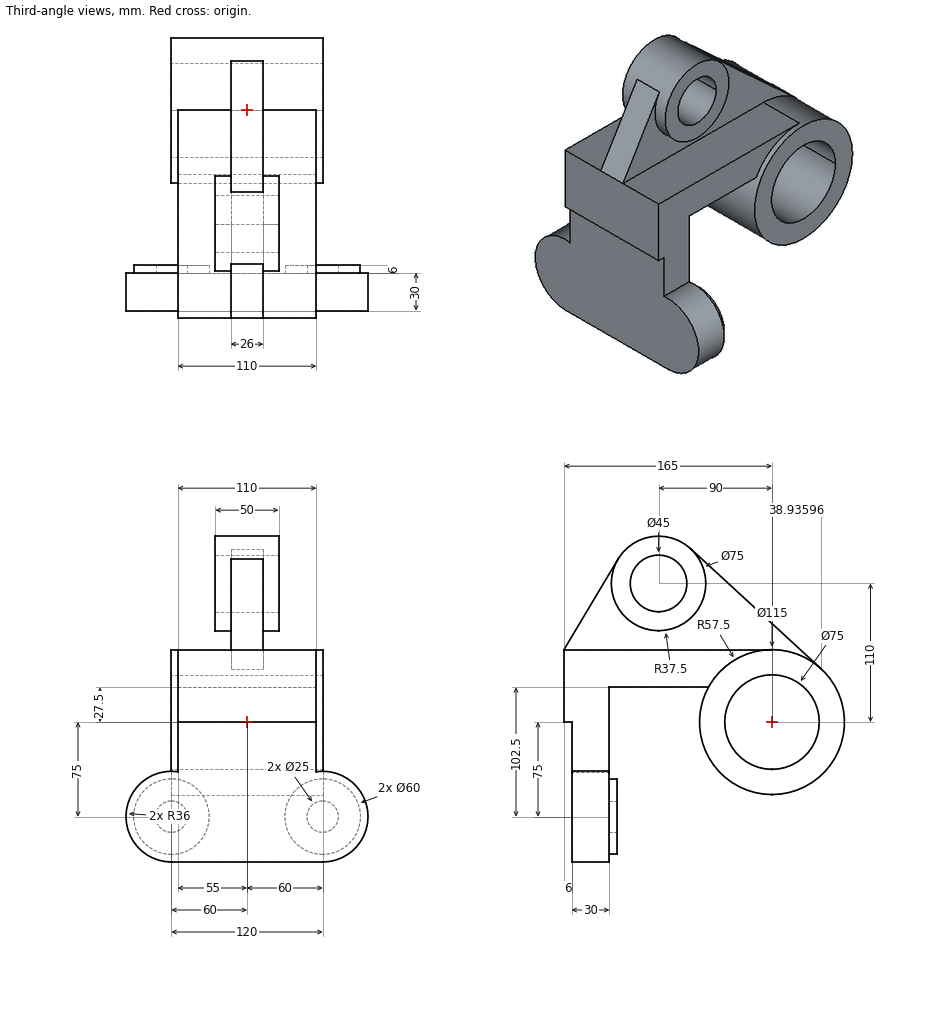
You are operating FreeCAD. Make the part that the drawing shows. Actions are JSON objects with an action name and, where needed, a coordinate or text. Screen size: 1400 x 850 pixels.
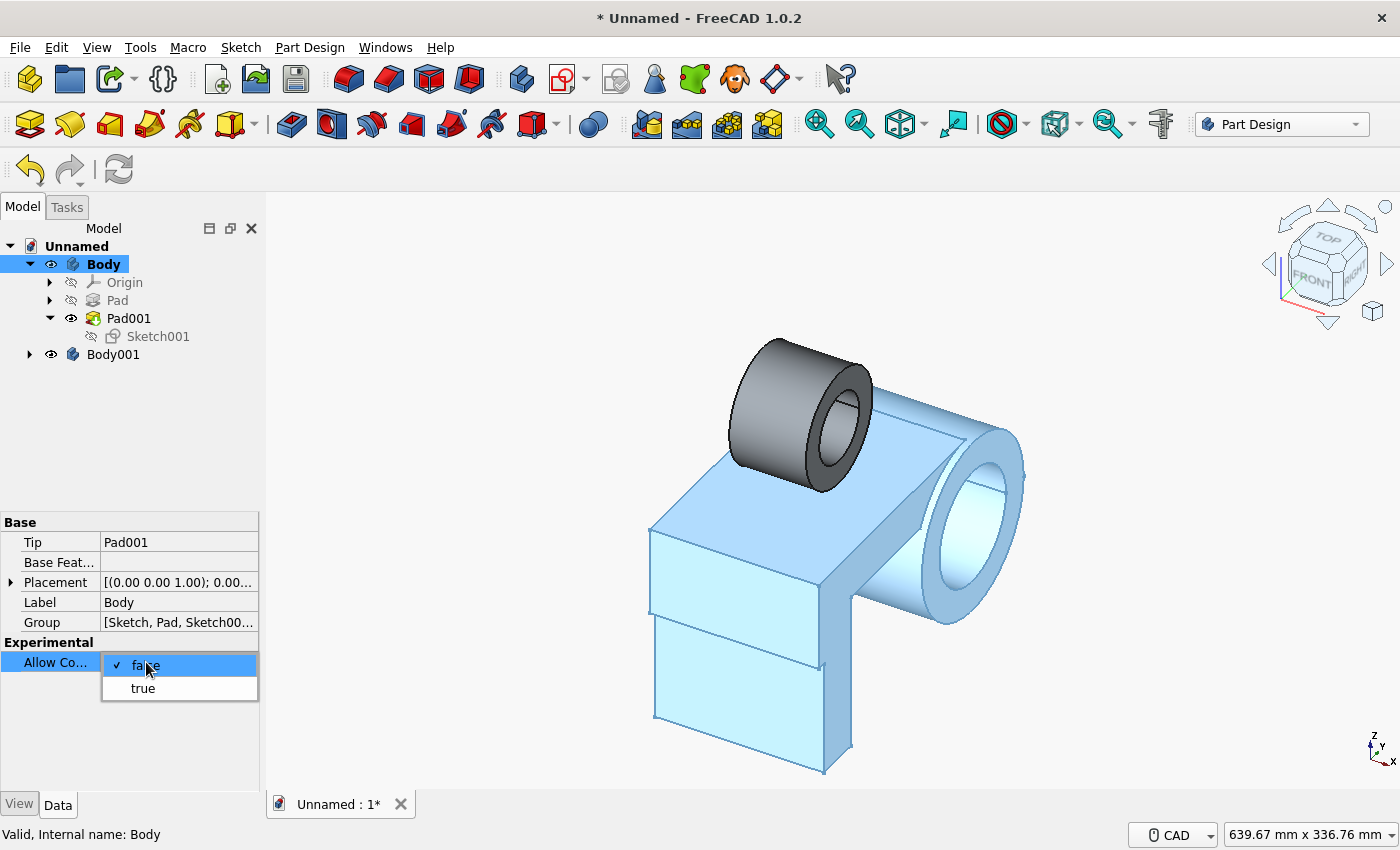
{"action": "left_click", "coordinate": [179, 688]}
{"action": "key", "text": "Return"}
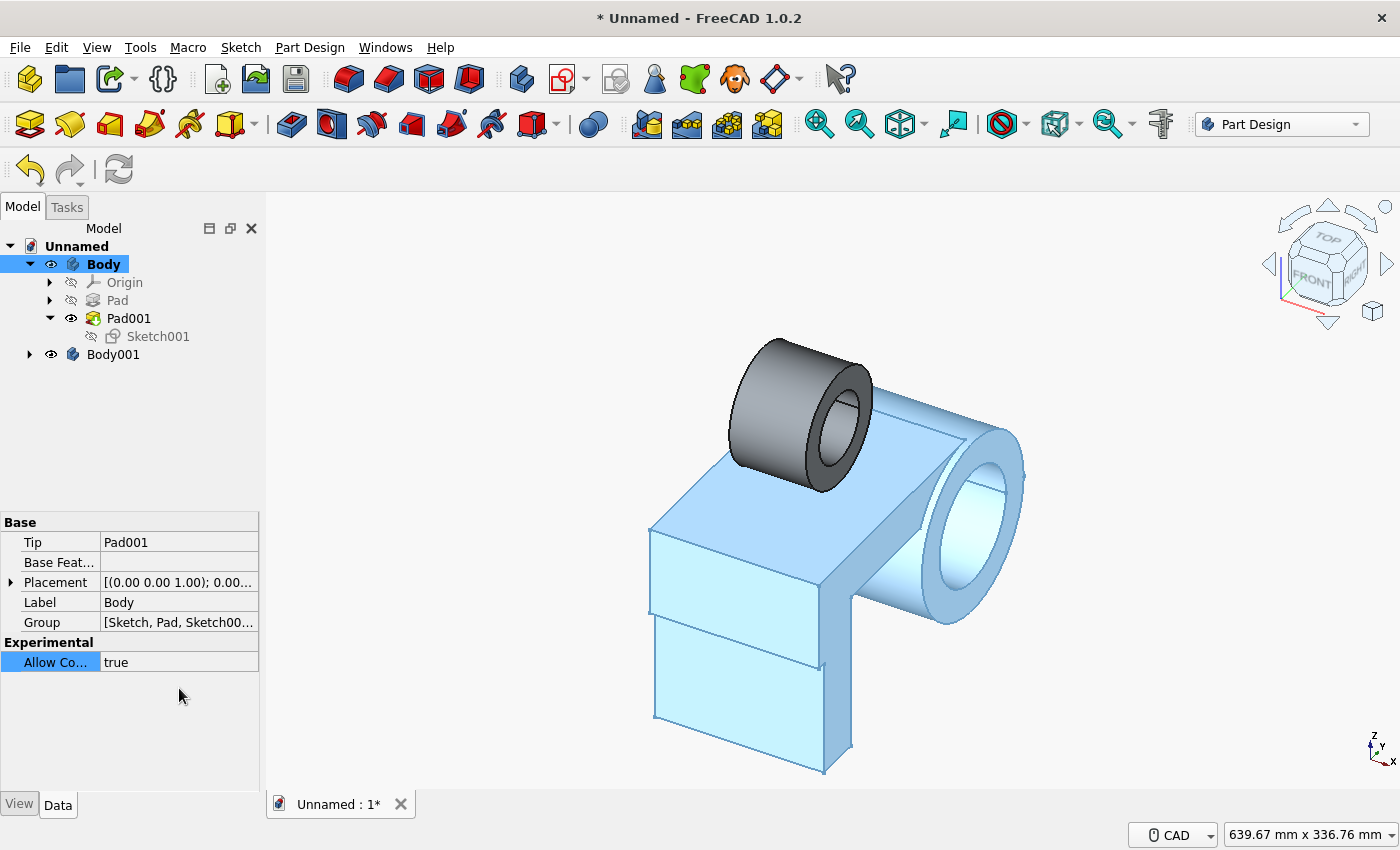
{"action": "left_click", "coordinate": [96, 354]}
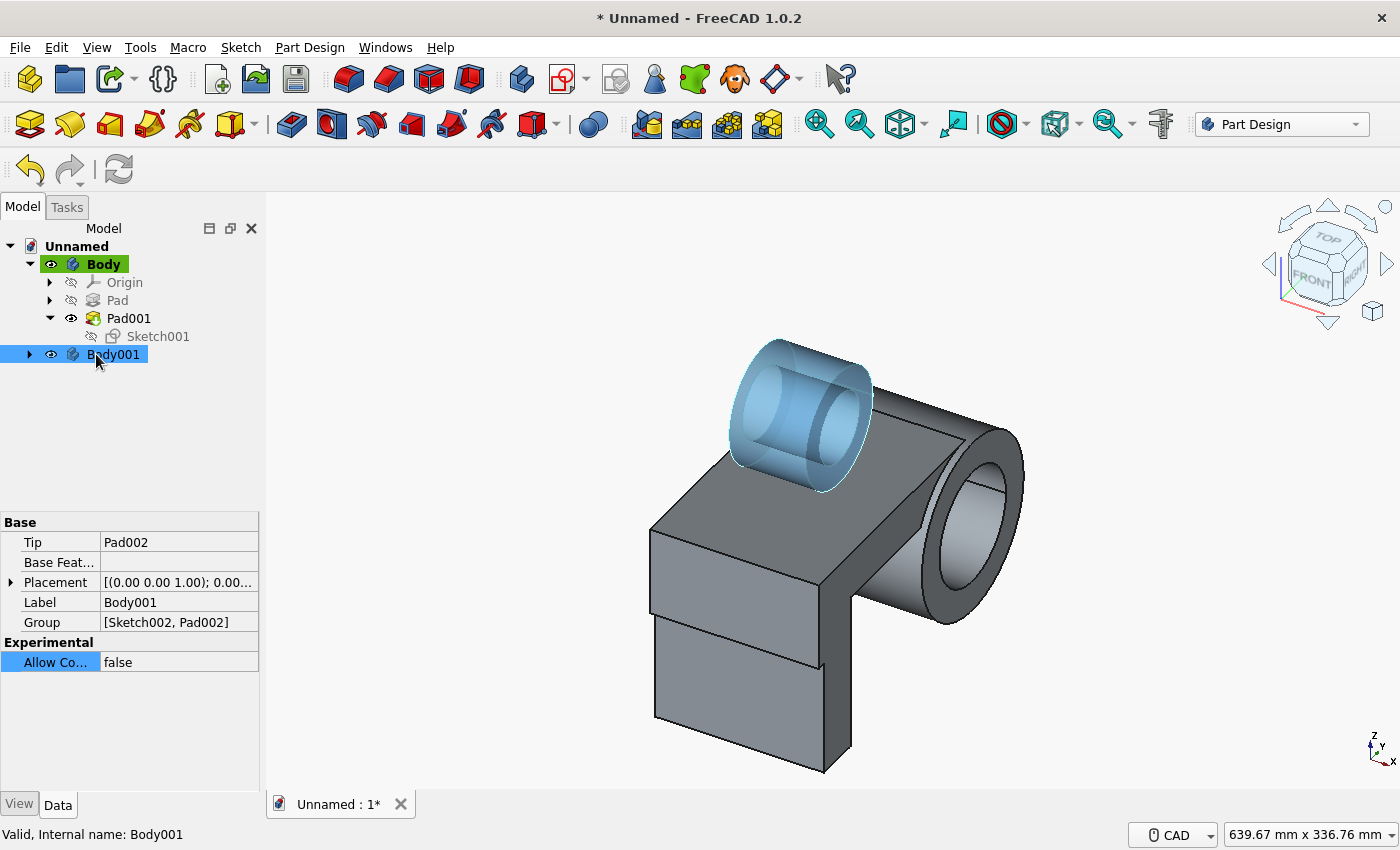
{"action": "left_click", "coordinate": [594, 124]}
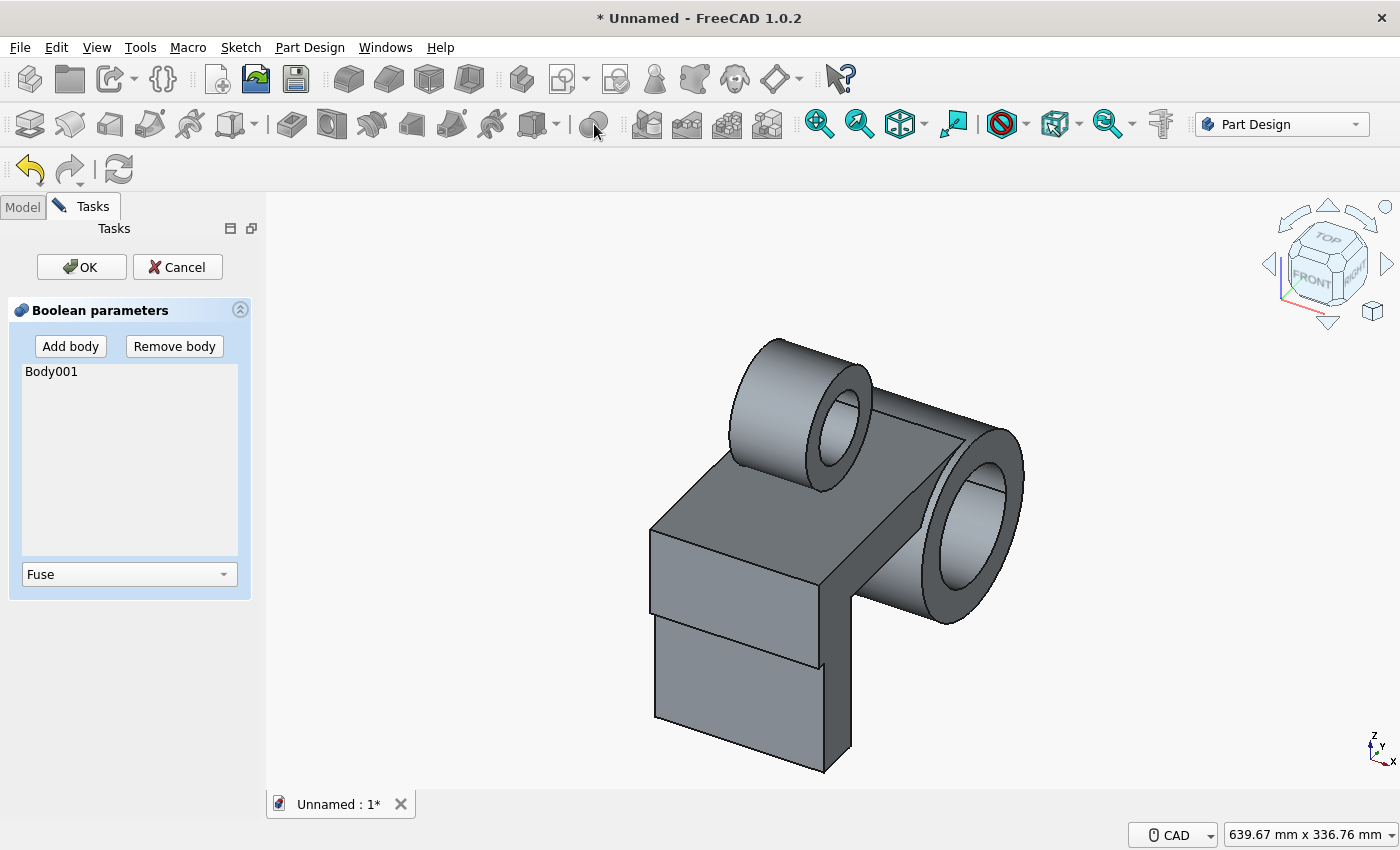
{"action": "left_click", "coordinate": [82, 267]}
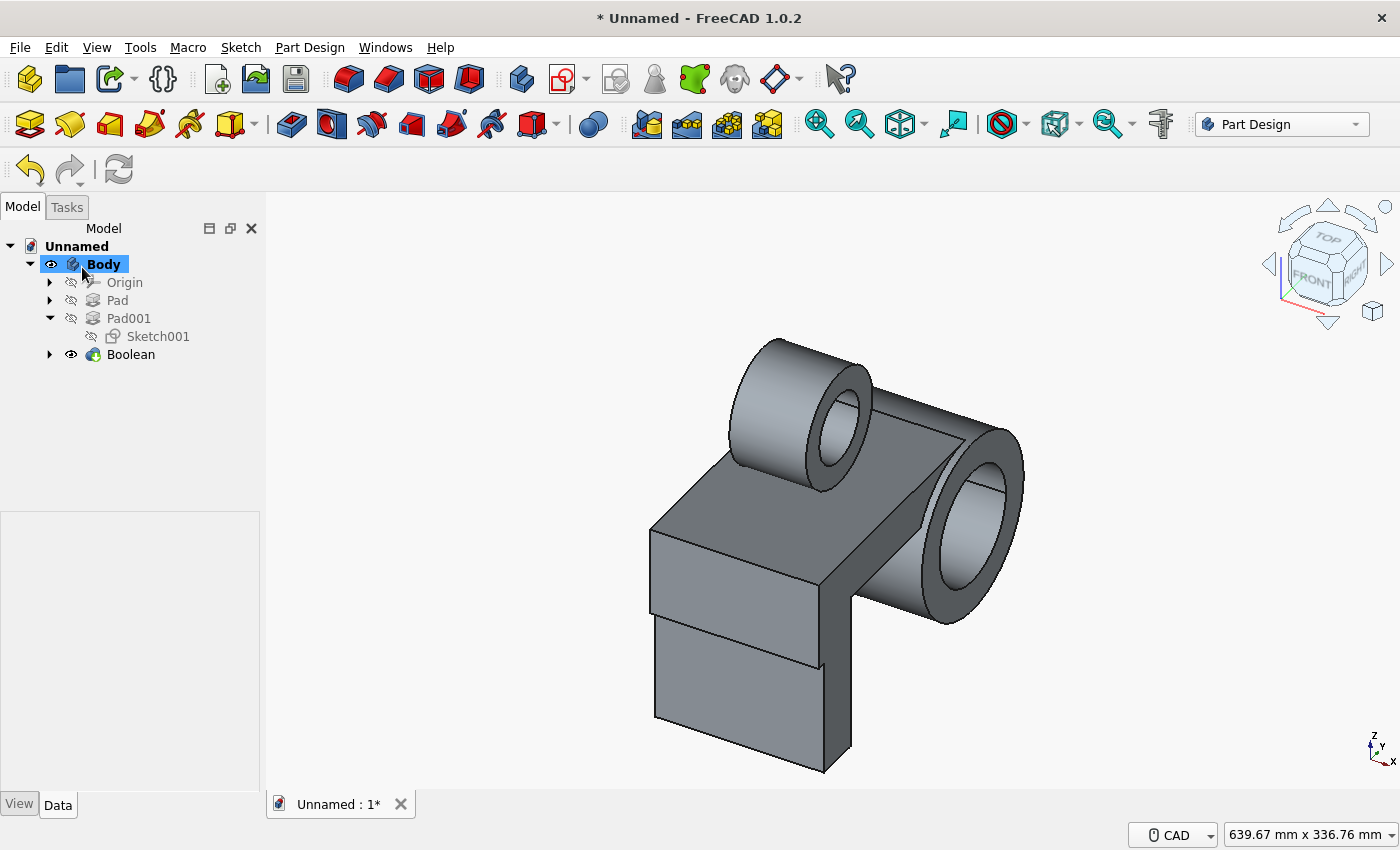
{"action": "left_click", "coordinate": [562, 80]}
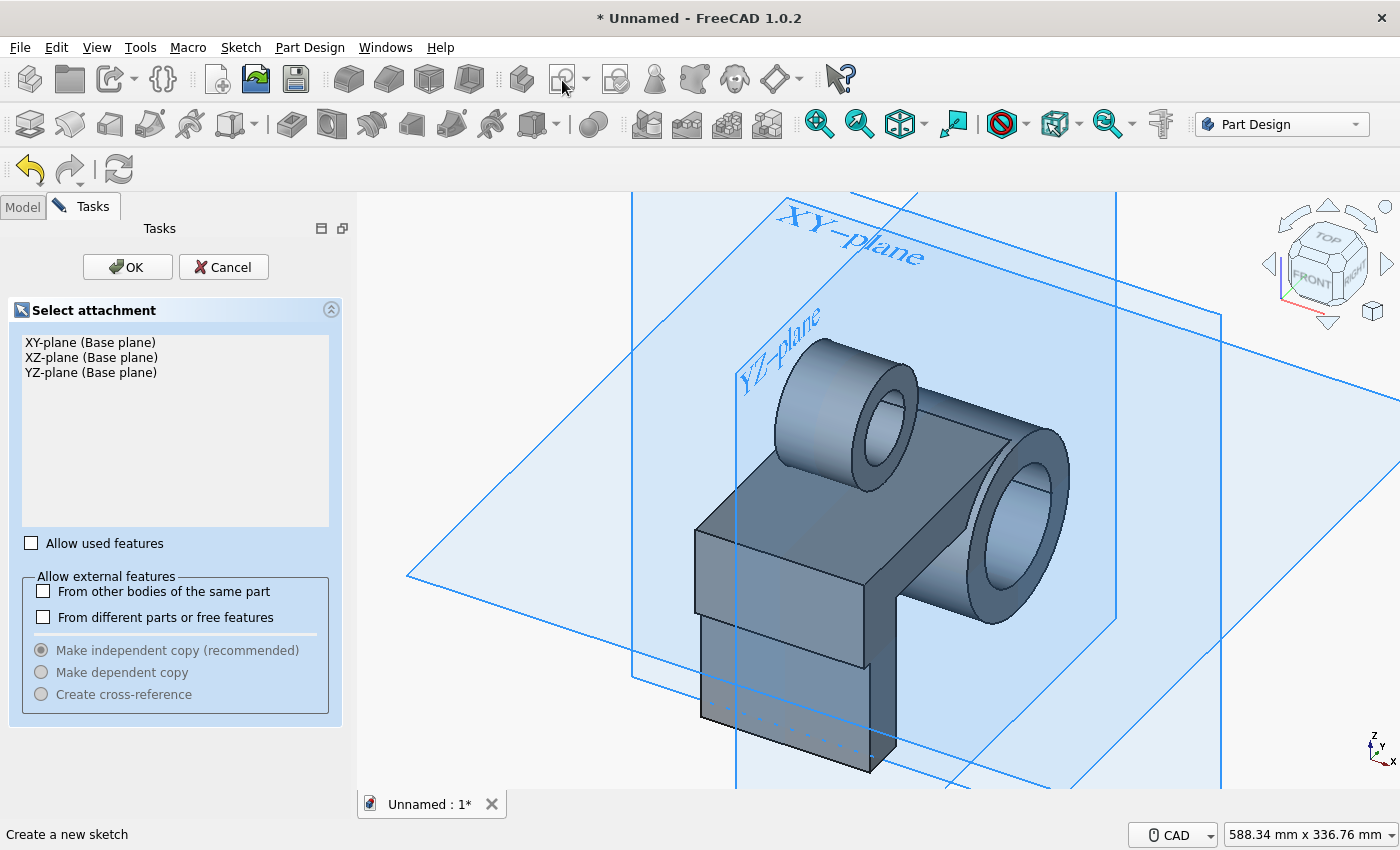
{"action": "left_click", "coordinate": [82, 372]}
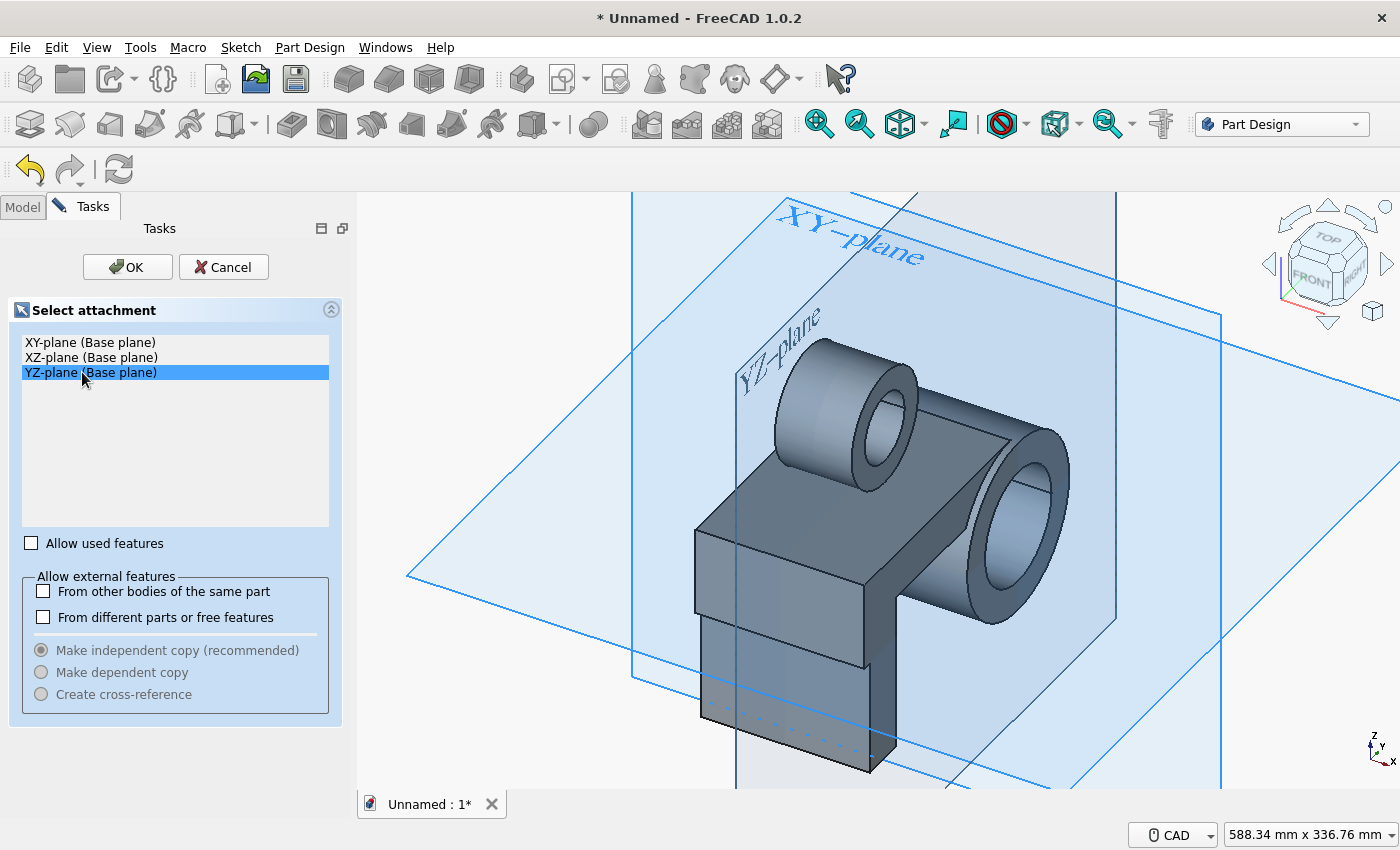
{"action": "left_click", "coordinate": [128, 267]}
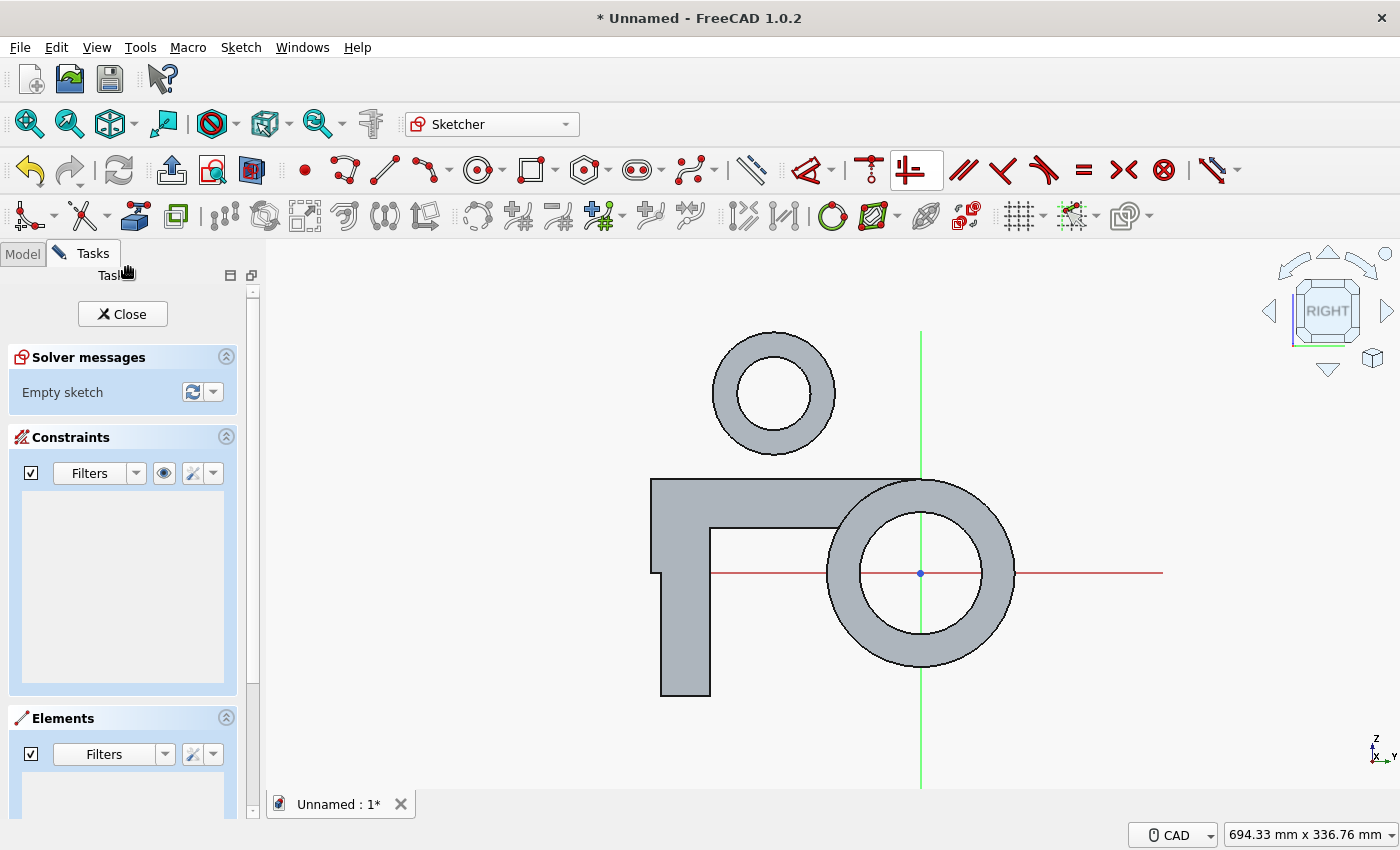
{"action": "left_click", "coordinate": [252, 170]}